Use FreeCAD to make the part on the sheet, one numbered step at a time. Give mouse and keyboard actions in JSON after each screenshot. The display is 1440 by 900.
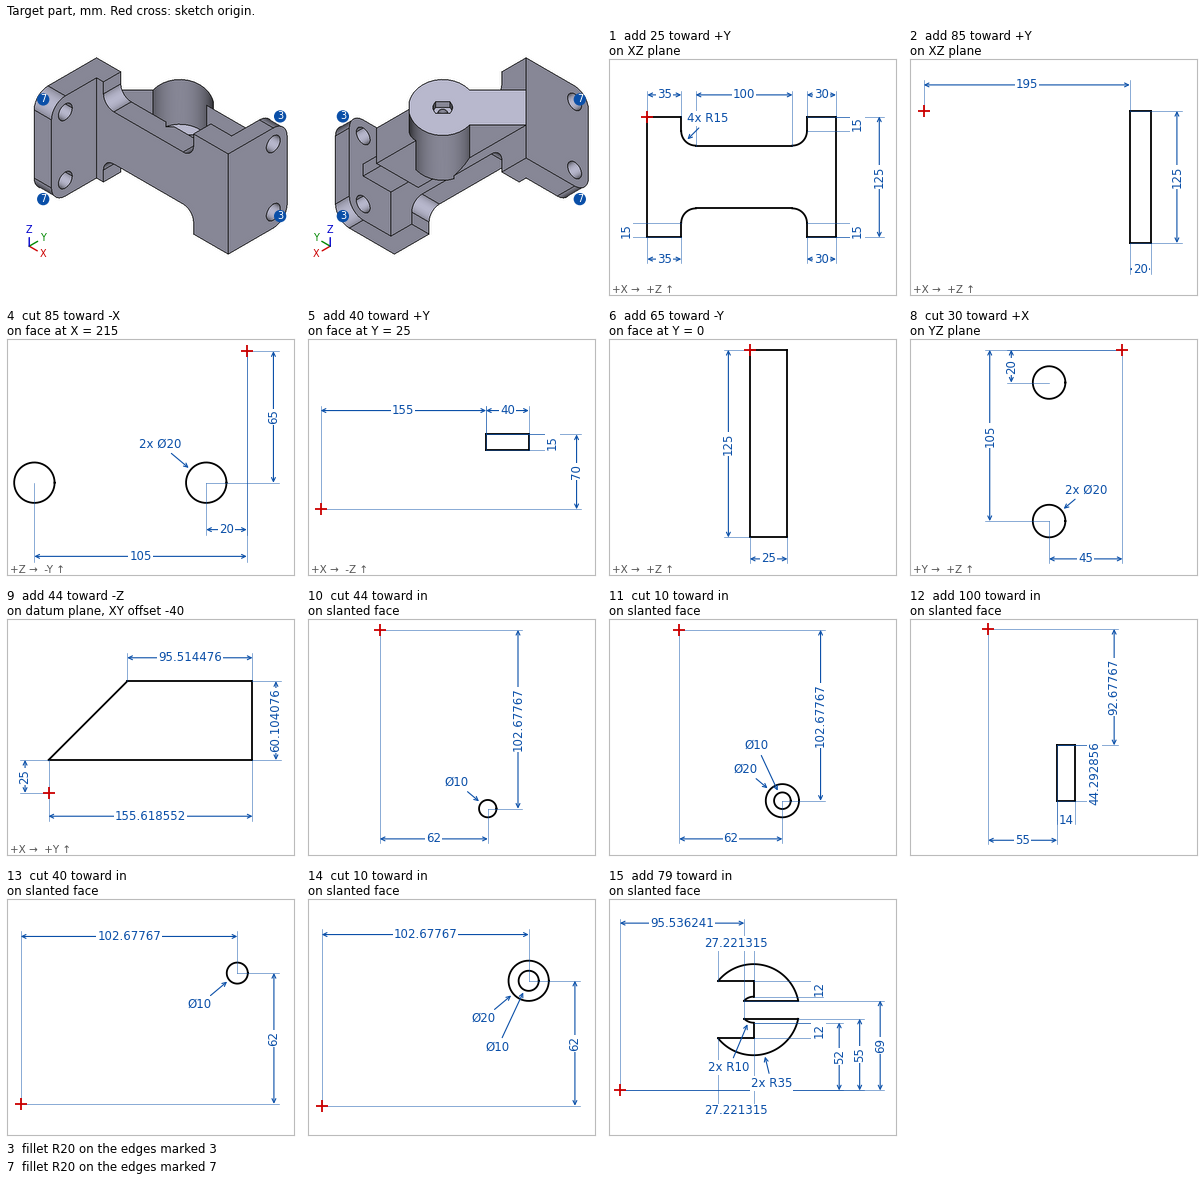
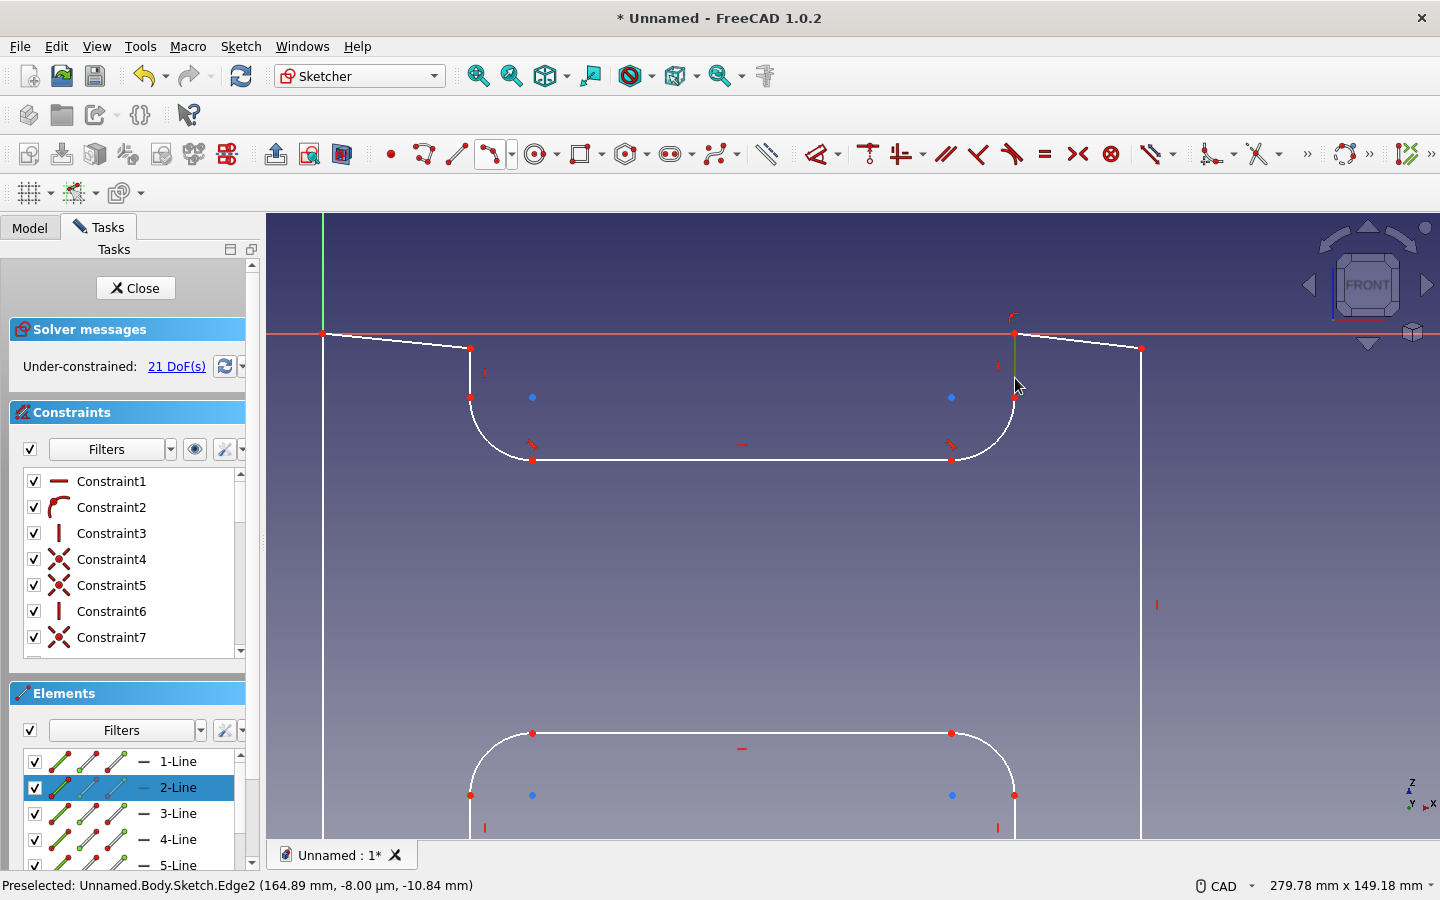
{"action": "left_click", "coordinate": [980, 453]}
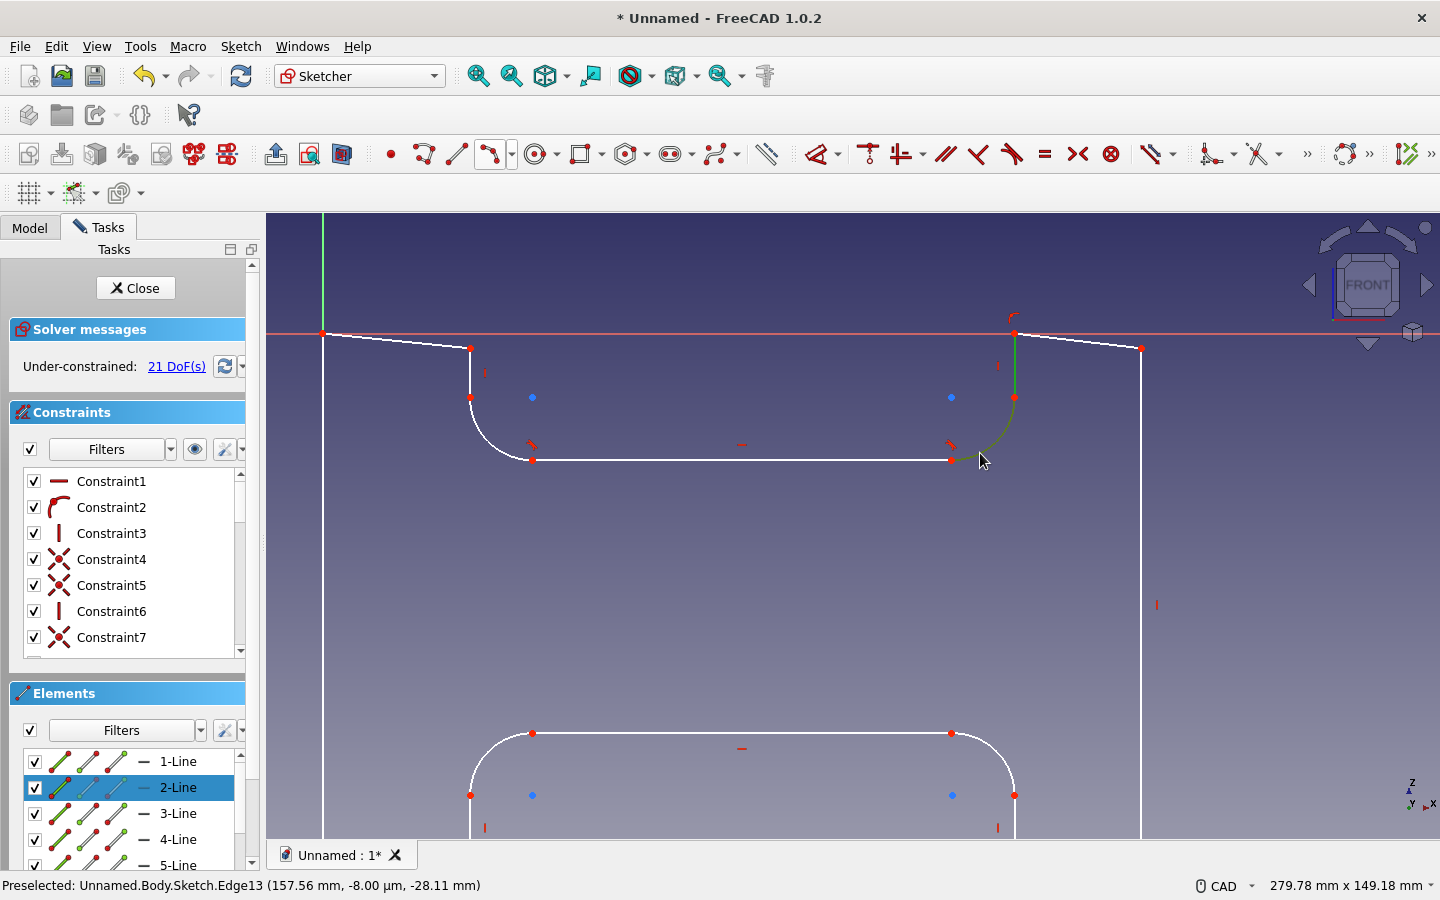
{"action": "left_click", "coordinate": [1012, 154]}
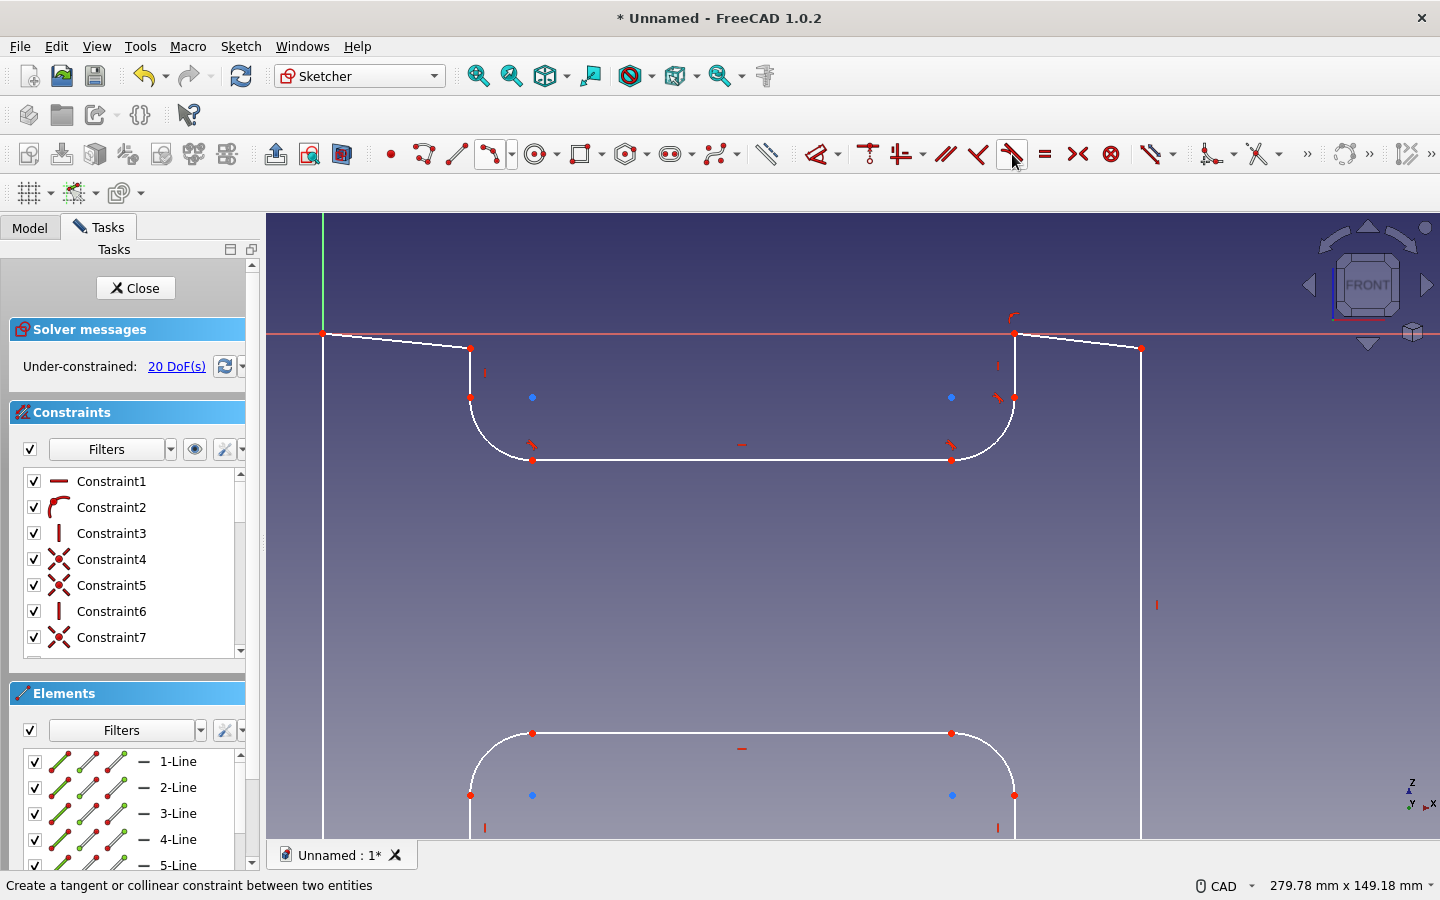
{"action": "left_click", "coordinate": [1015, 809]}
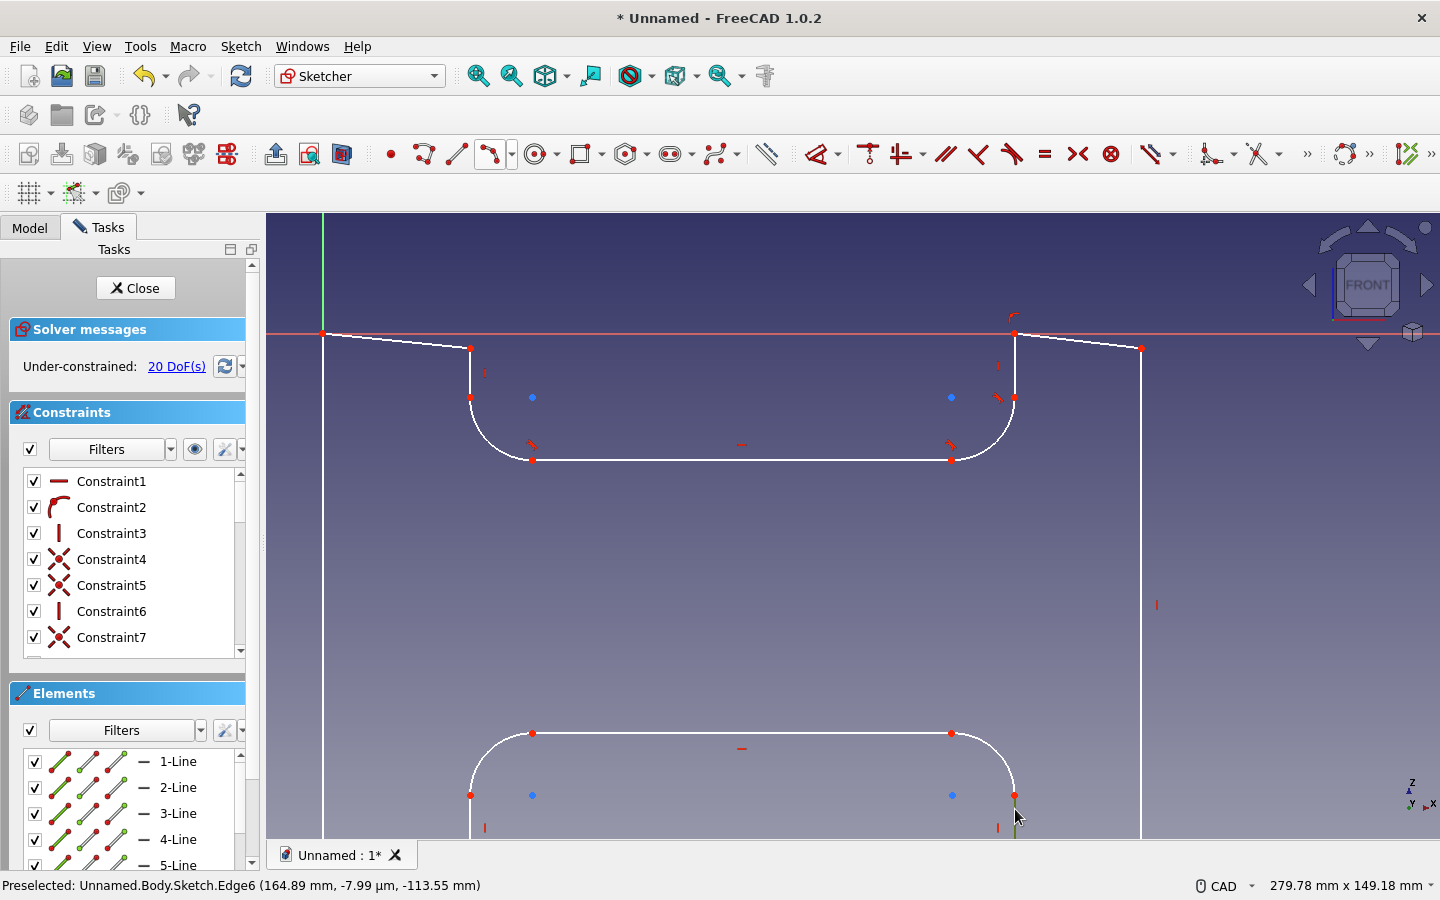
{"action": "left_click", "coordinate": [1008, 767]}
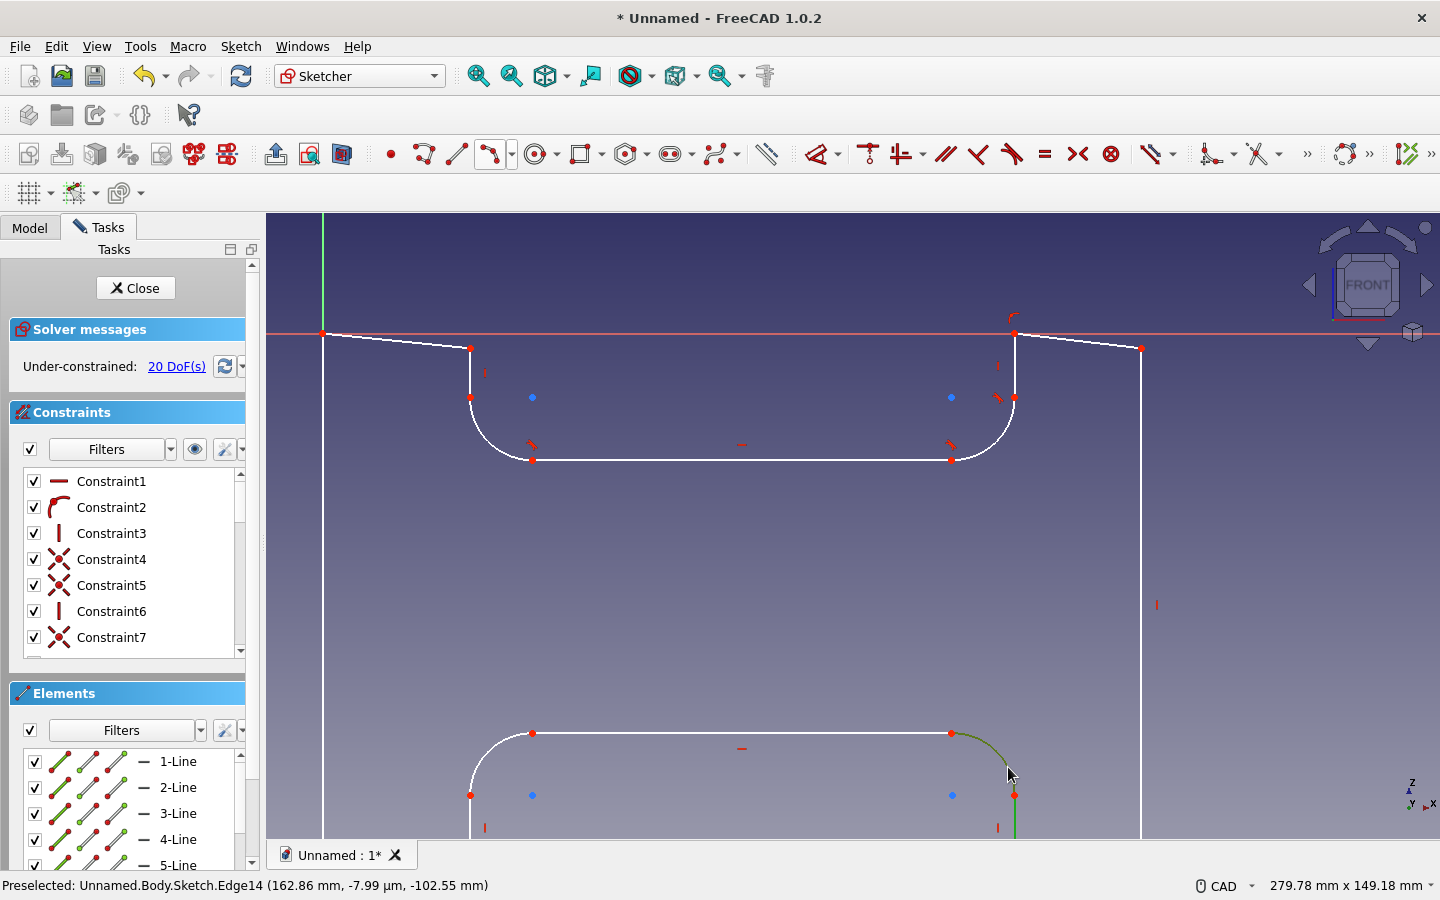
{"action": "left_click", "coordinate": [1012, 154]}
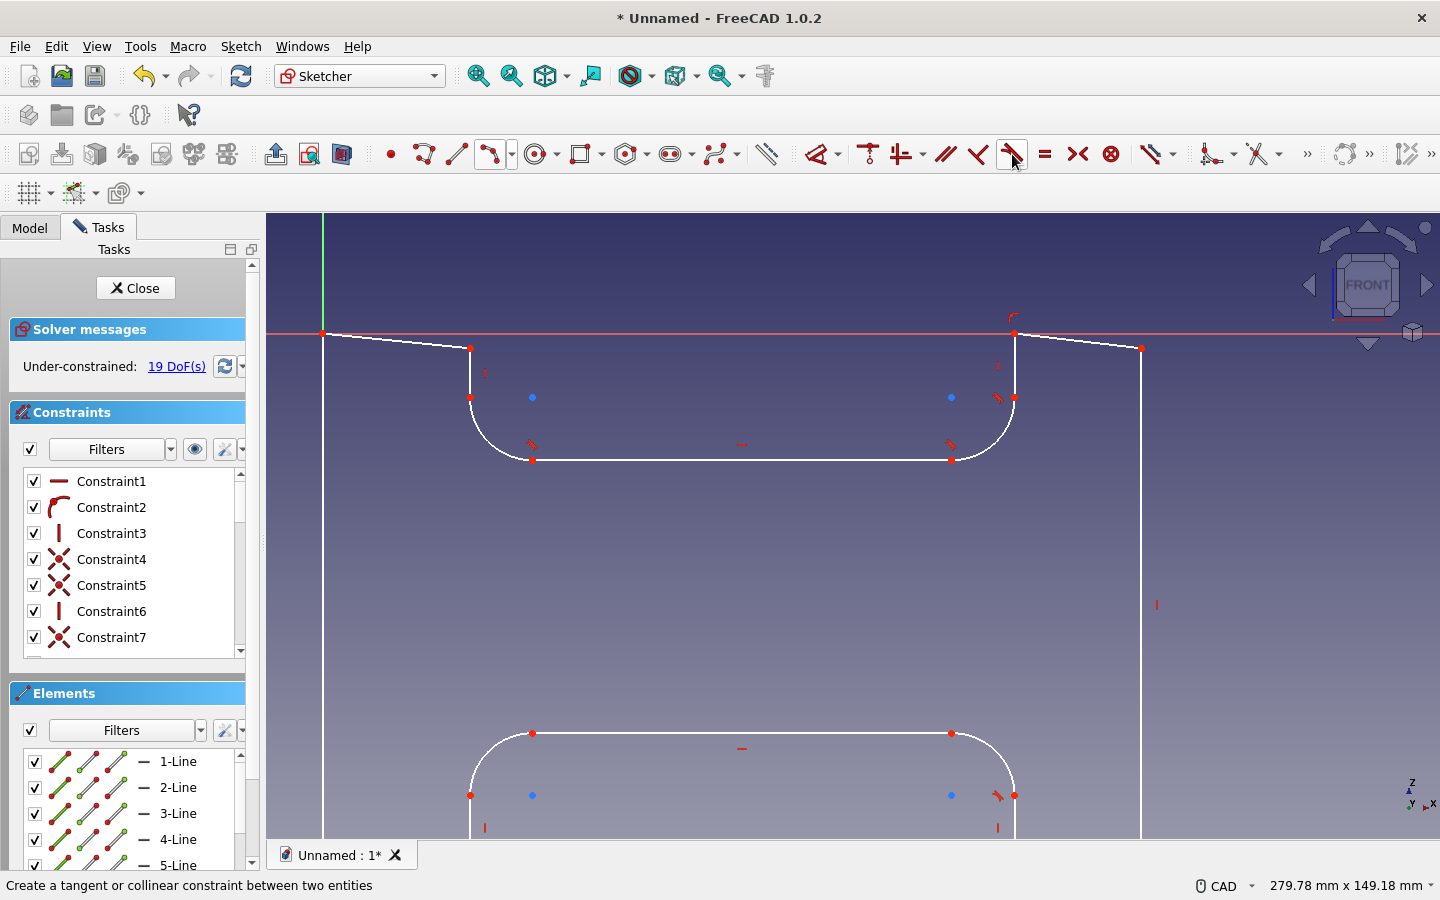
{"action": "left_click", "coordinate": [826, 733]}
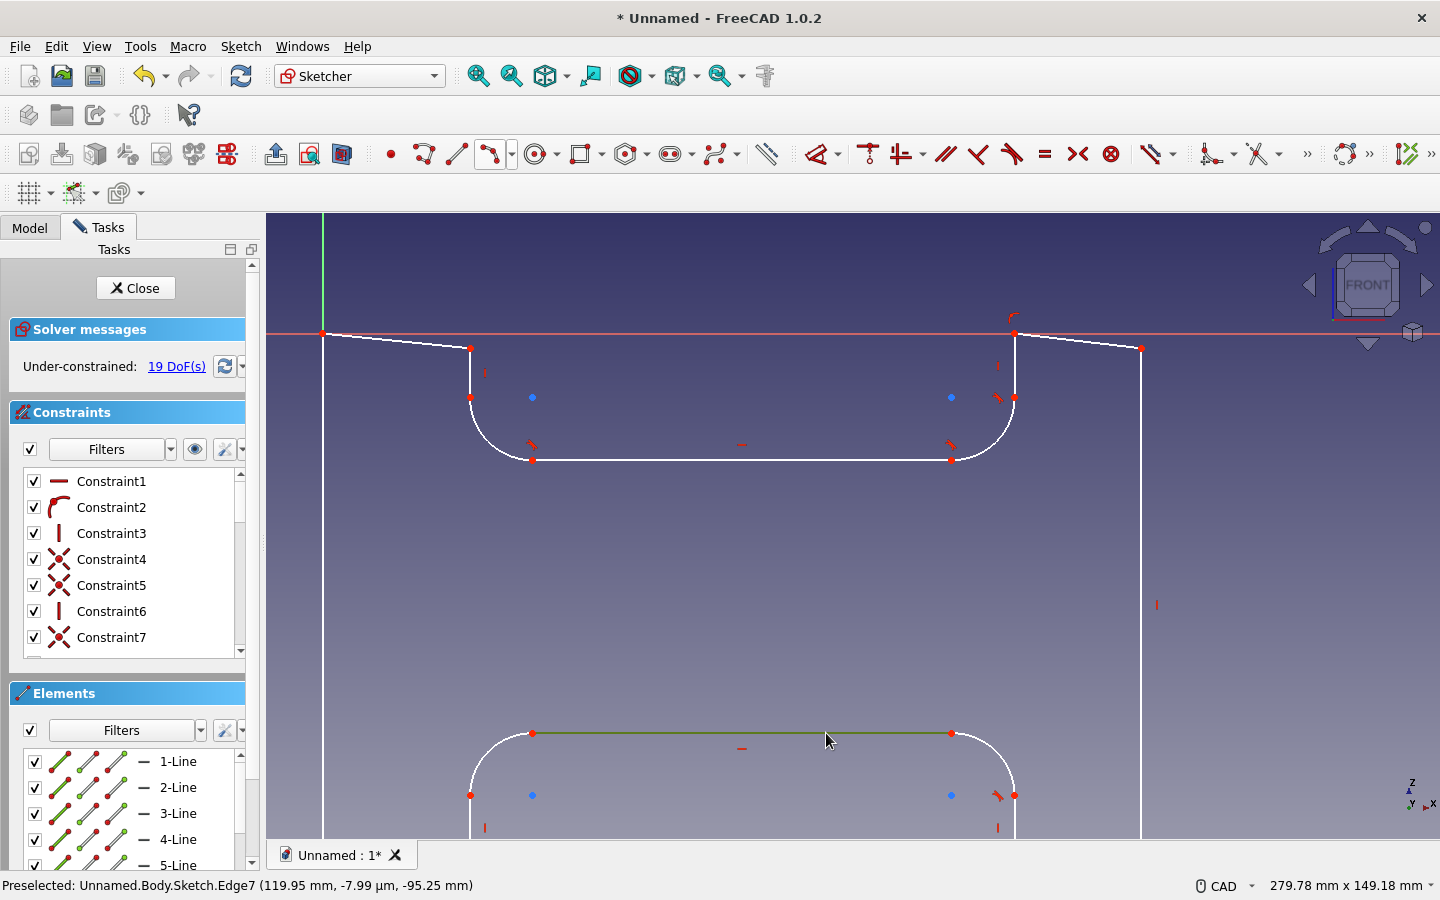
{"action": "left_click", "coordinate": [1008, 767]}